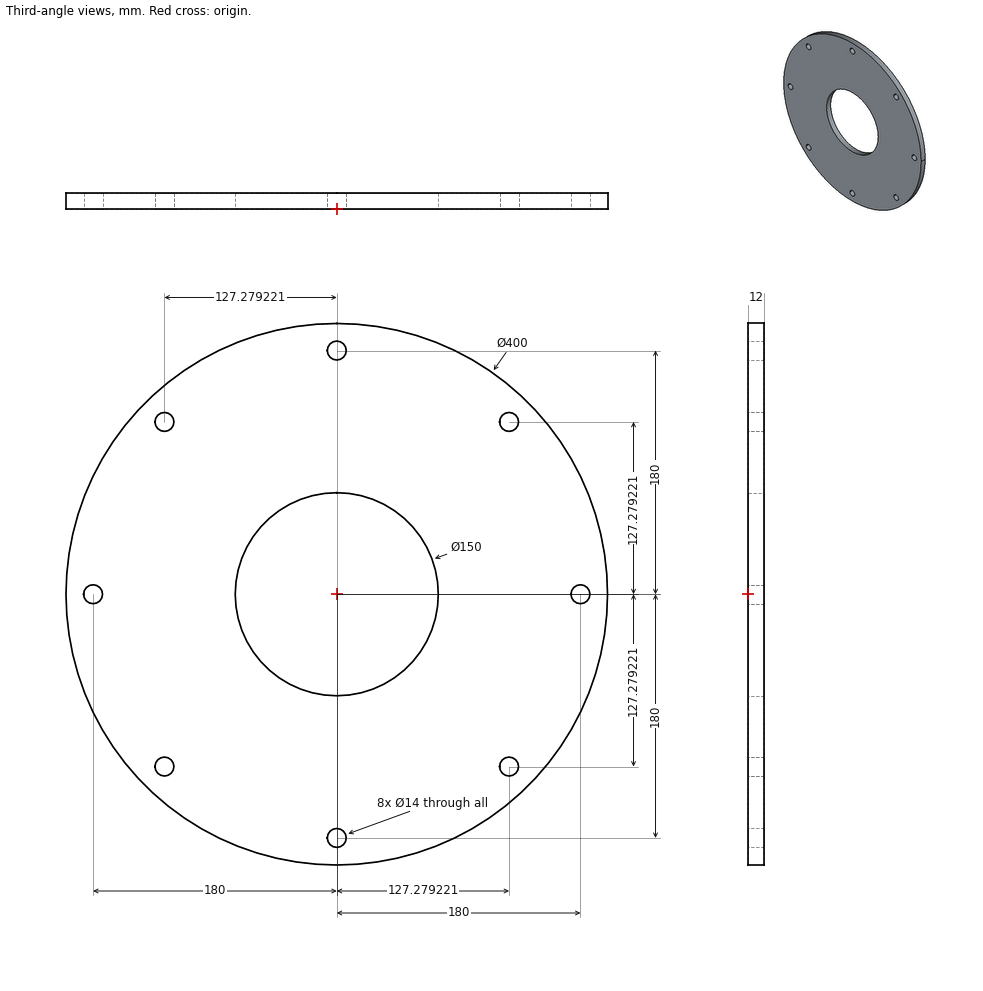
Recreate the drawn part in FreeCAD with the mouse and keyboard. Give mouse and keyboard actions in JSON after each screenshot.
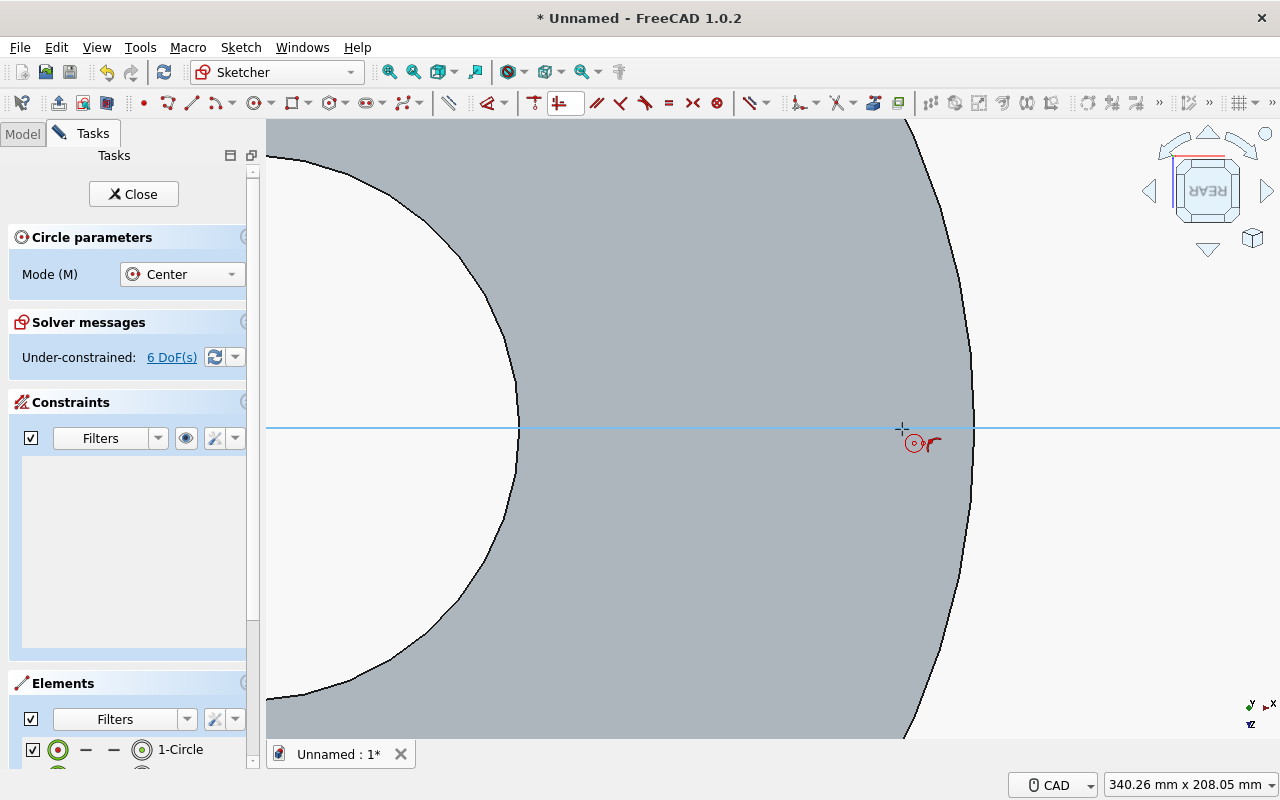
{"action": "left_click", "coordinate": [902, 428]}
{"action": "left_click", "coordinate": [920, 410]}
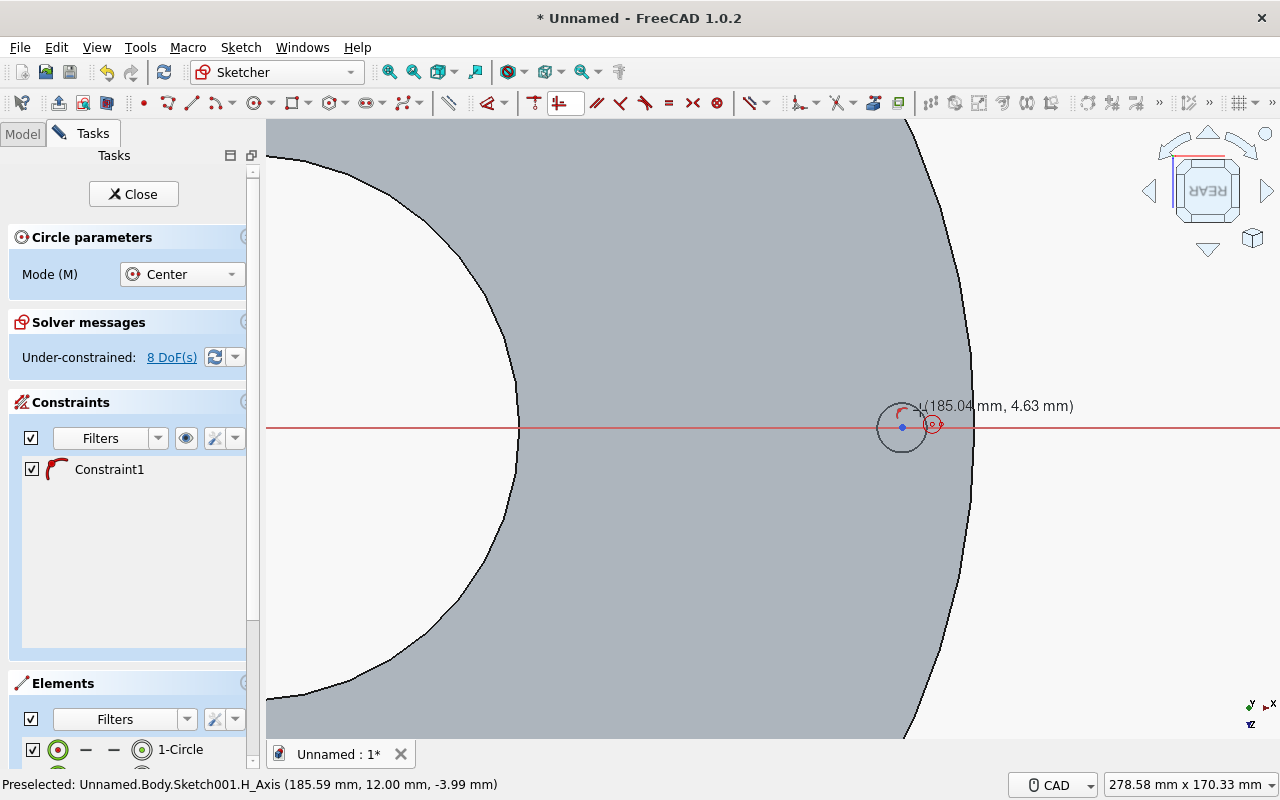
{"action": "scroll", "coordinate": [902, 430], "scroll_direction": "down", "scroll_amount": 6}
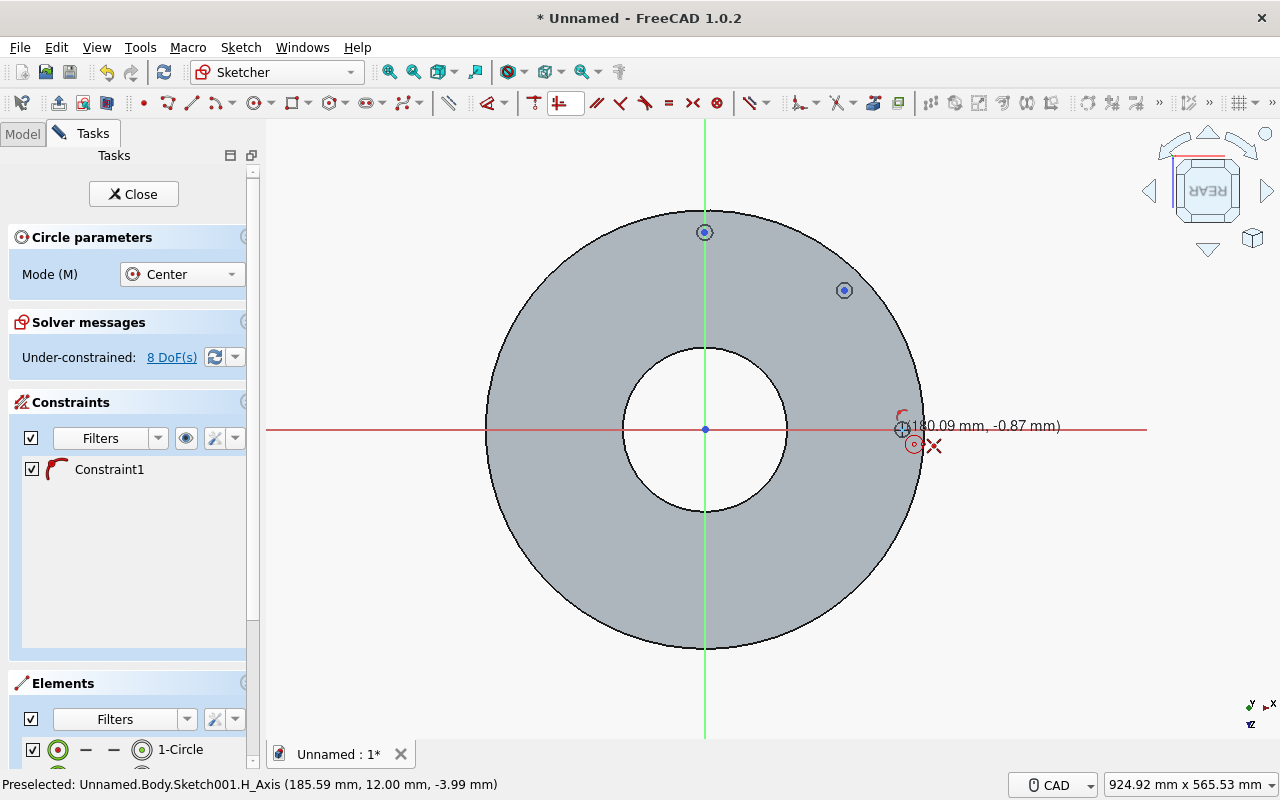
{"action": "scroll", "coordinate": [845, 569], "scroll_direction": "up", "scroll_amount": 6}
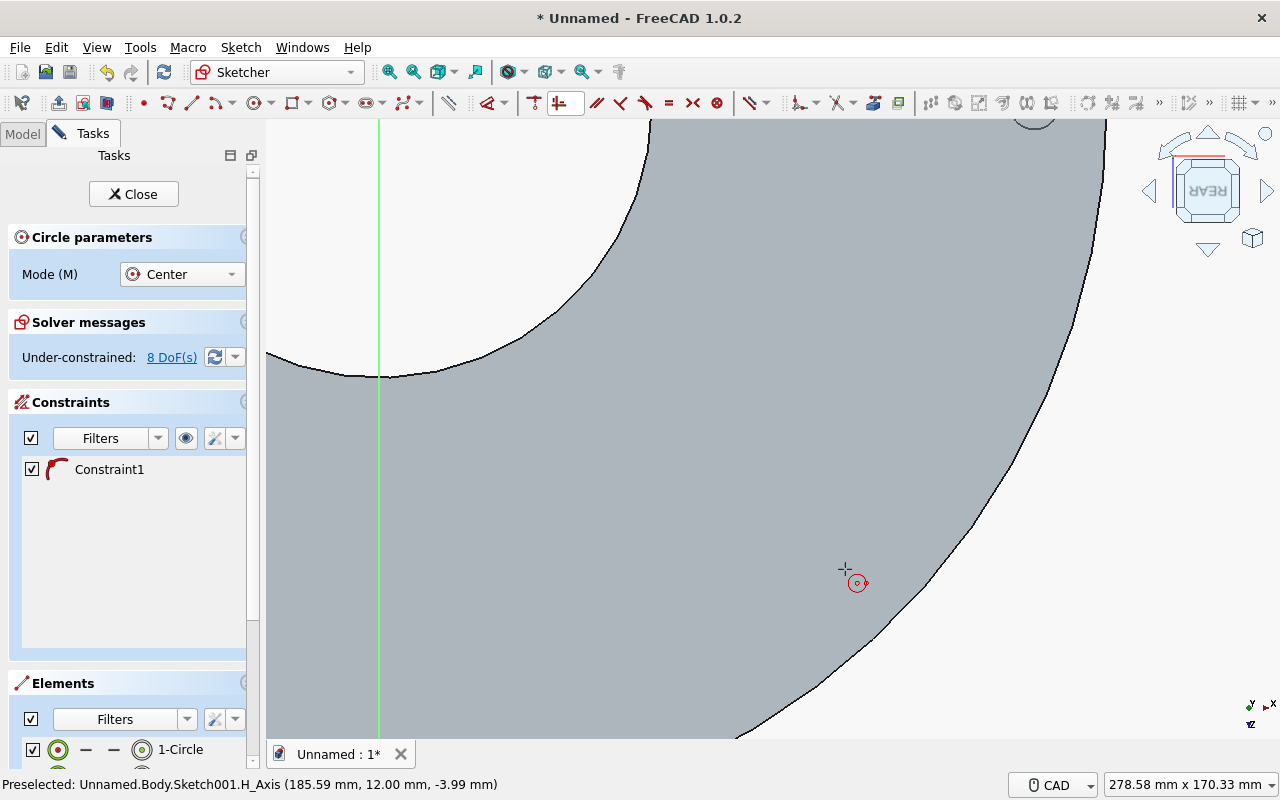
{"action": "left_click", "coordinate": [842, 568]}
{"action": "left_click", "coordinate": [860, 550]}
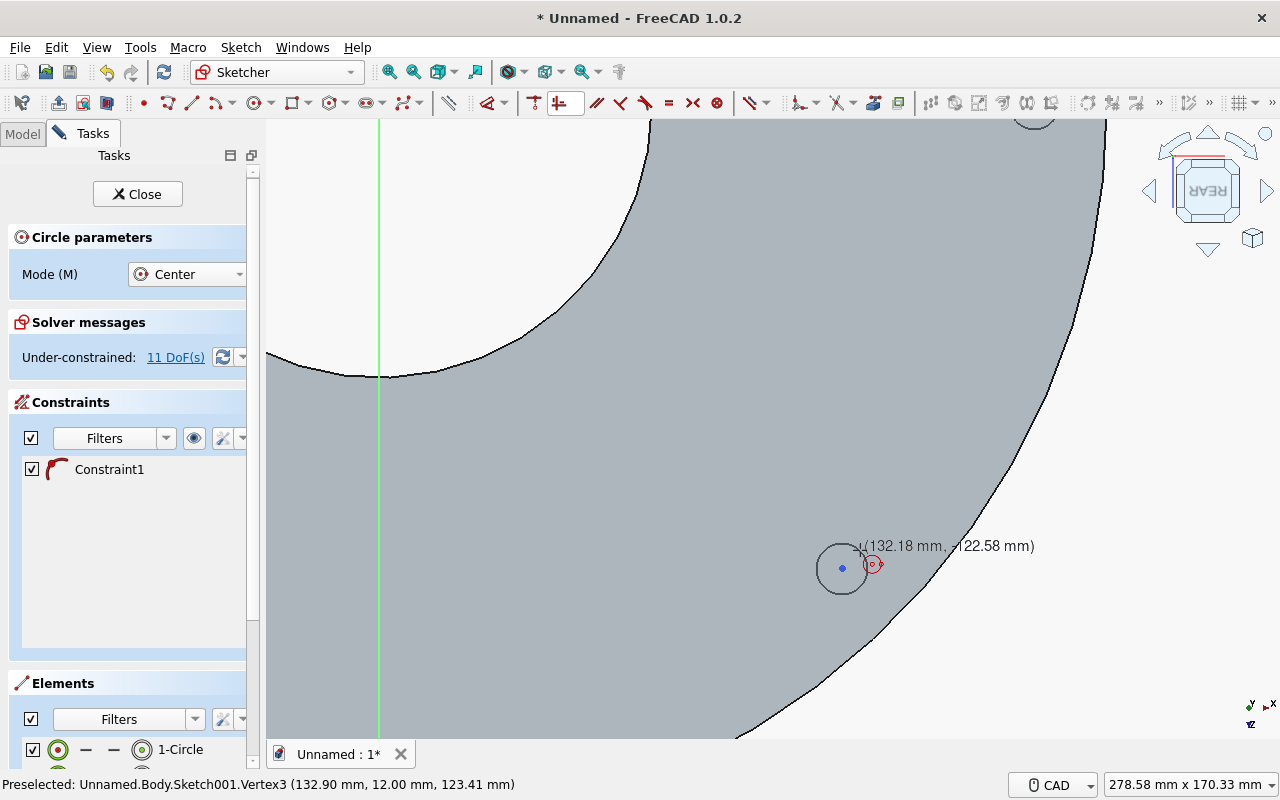
{"action": "scroll", "coordinate": [845, 569], "scroll_direction": "down", "scroll_amount": 6}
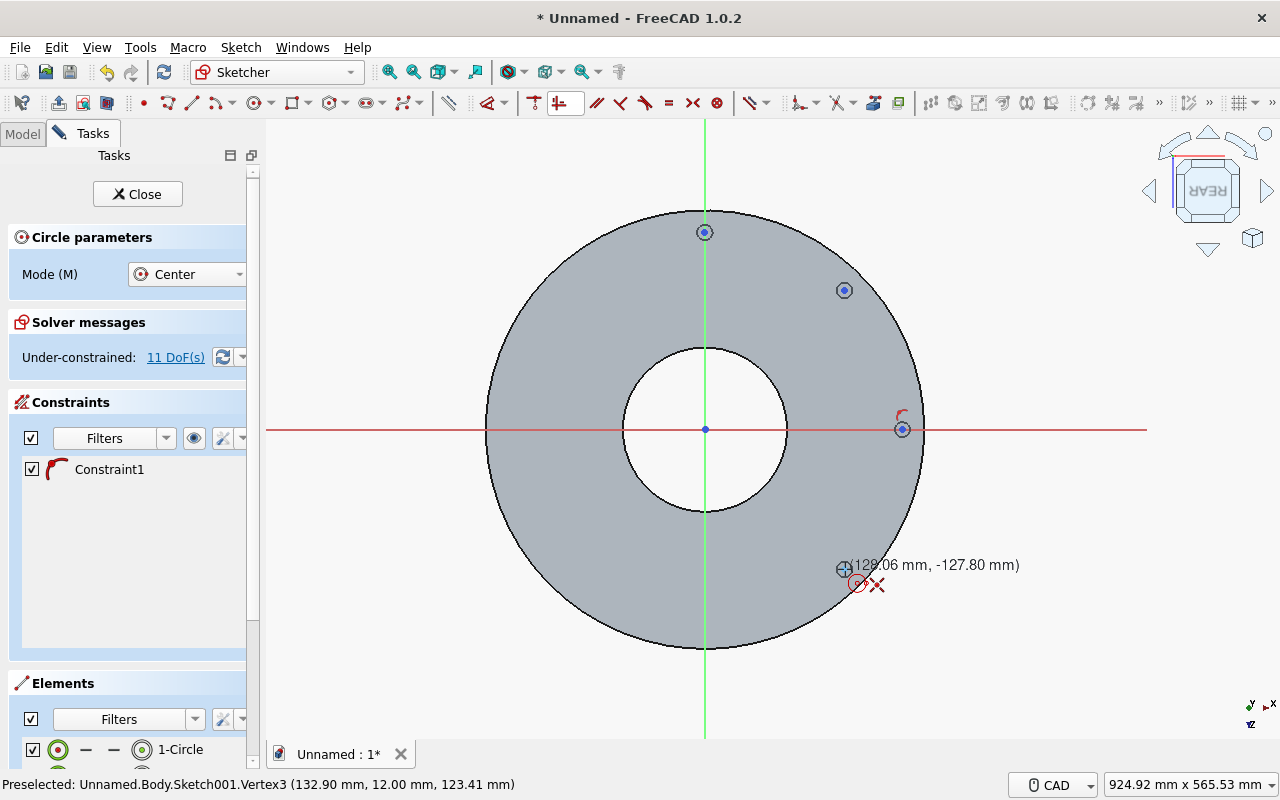
{"action": "scroll", "coordinate": [705, 627], "scroll_direction": "up", "scroll_amount": 6}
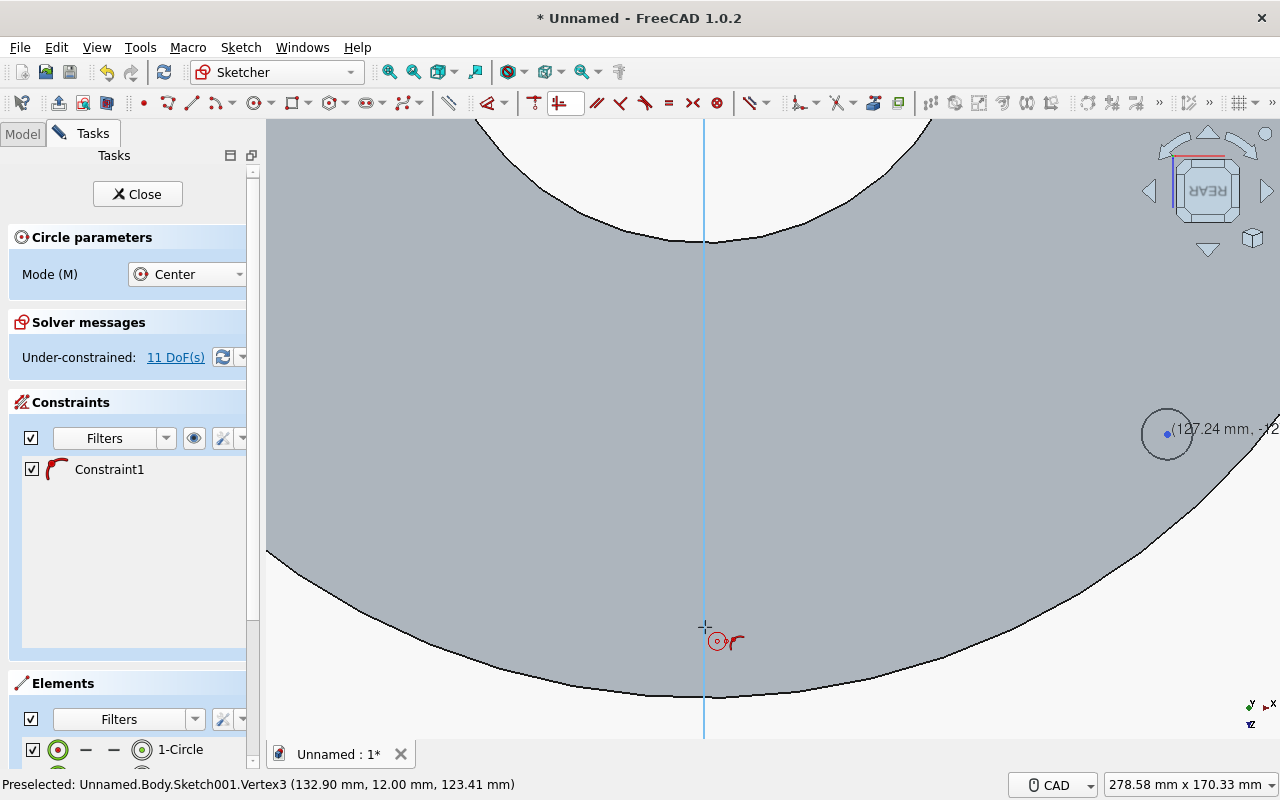
{"action": "left_click", "coordinate": [704, 625]}
{"action": "left_click", "coordinate": [722, 607]}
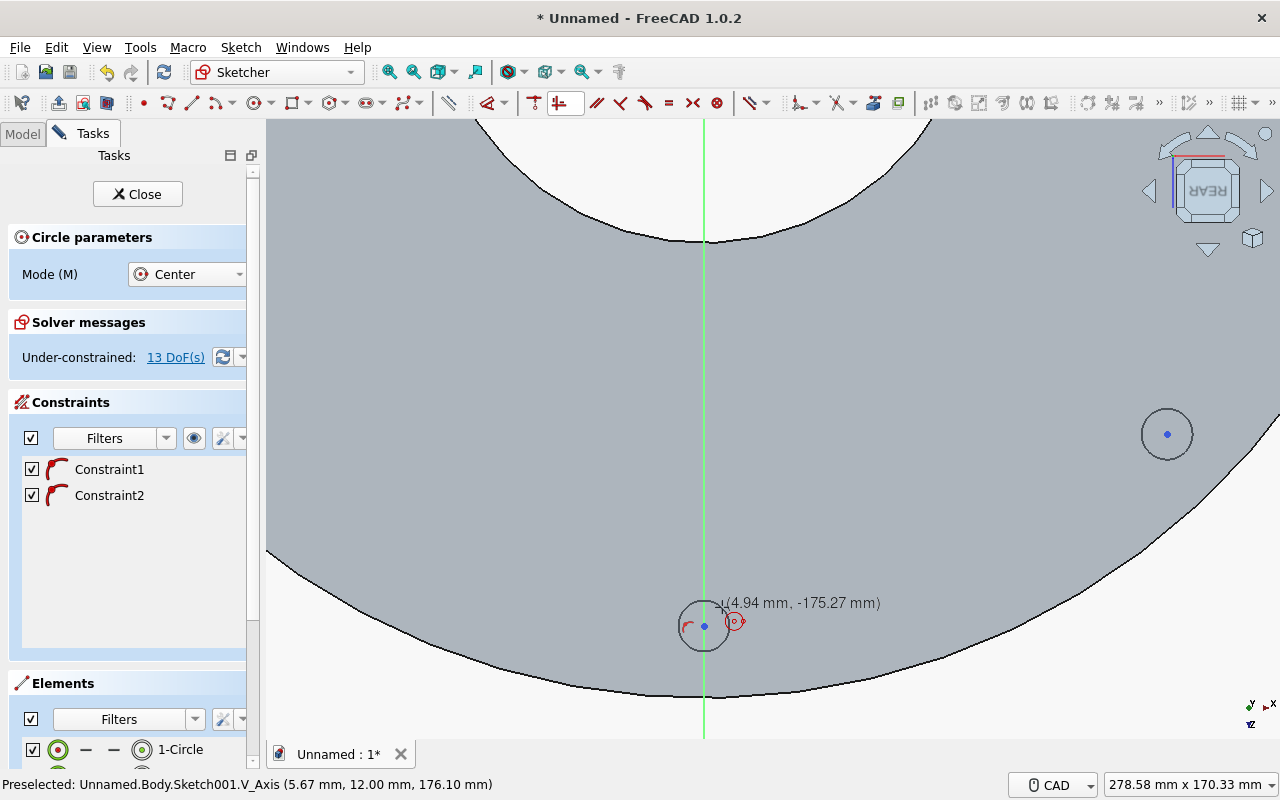
{"action": "scroll", "coordinate": [705, 627], "scroll_direction": "down", "scroll_amount": 6}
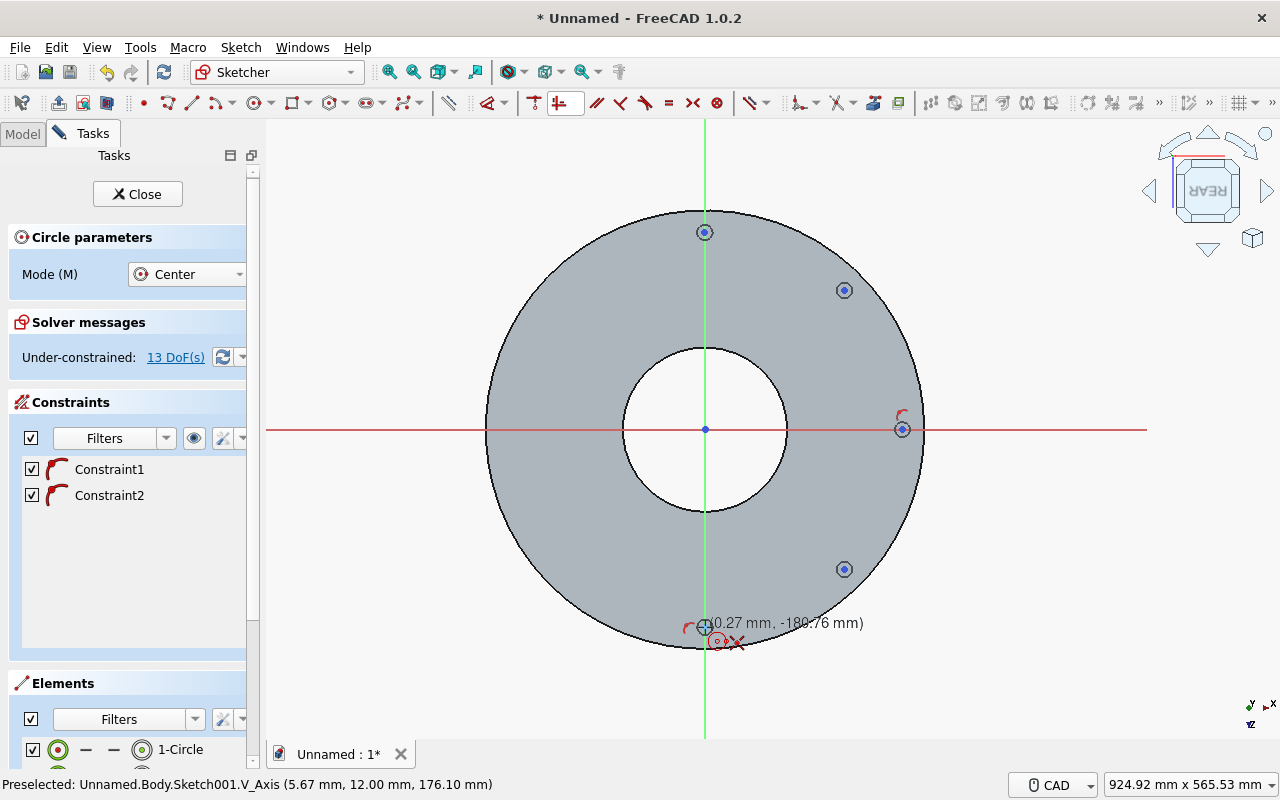
{"action": "scroll", "coordinate": [565, 569], "scroll_direction": "up", "scroll_amount": 6}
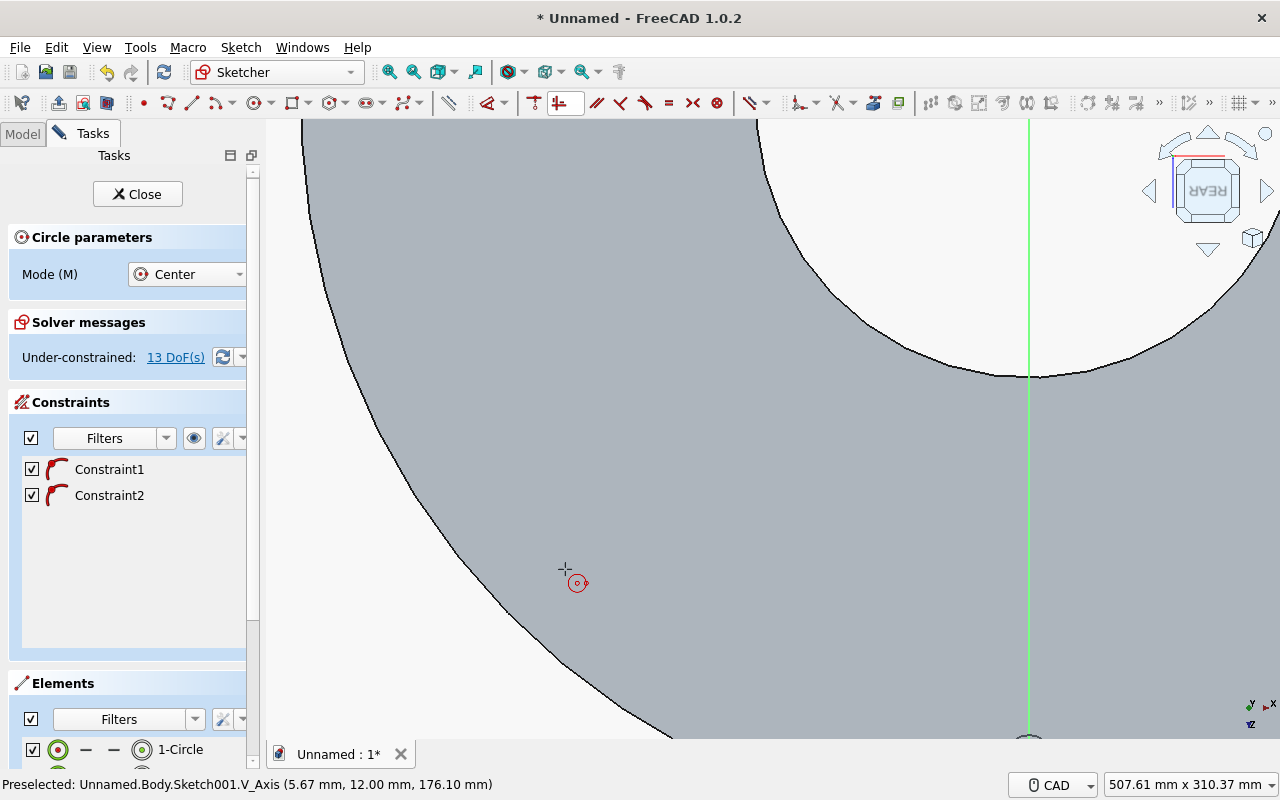
{"action": "left_click", "coordinate": [566, 568]}
{"action": "left_click", "coordinate": [584, 550]}